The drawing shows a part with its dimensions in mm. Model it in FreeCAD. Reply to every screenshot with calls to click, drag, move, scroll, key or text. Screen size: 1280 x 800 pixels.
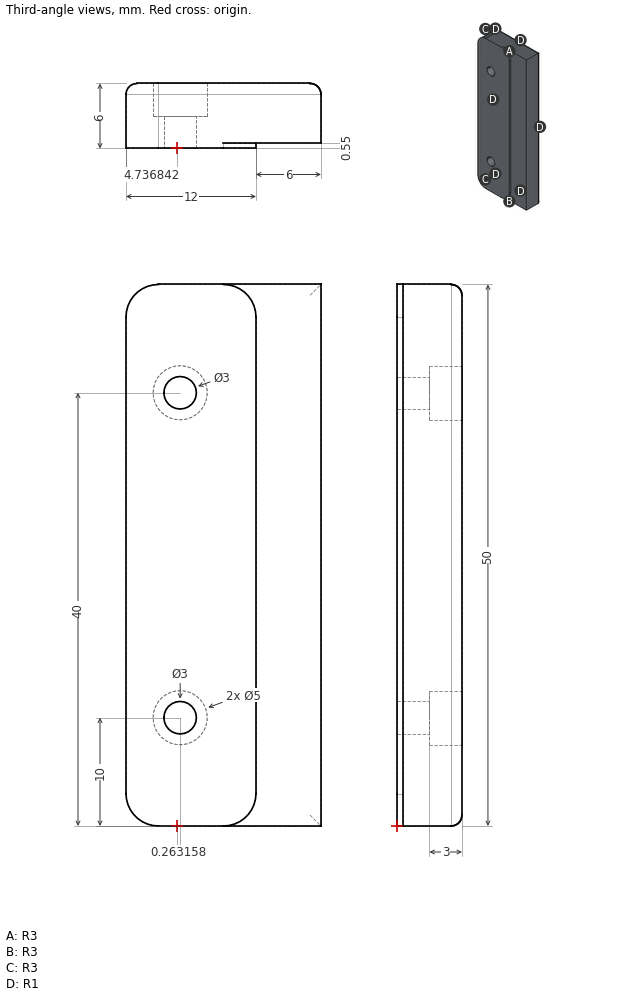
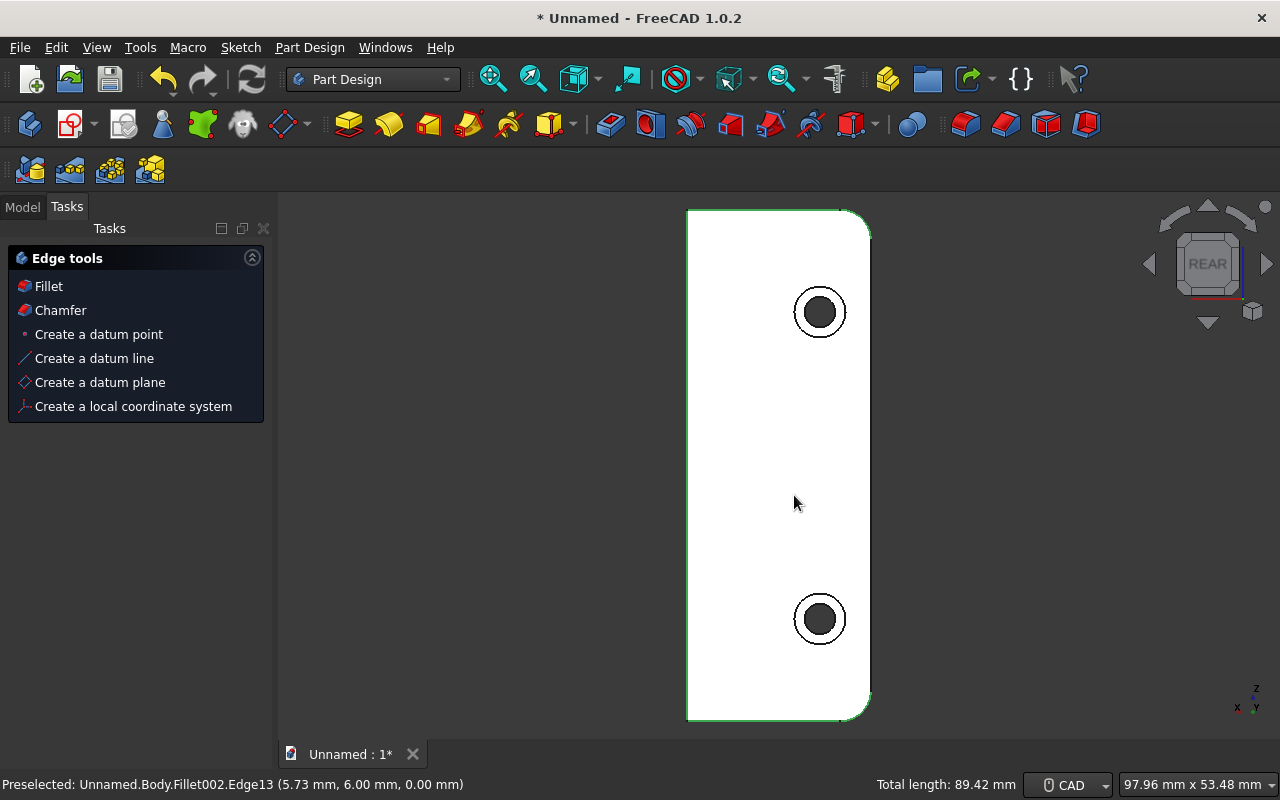
click(871, 464, ctrl)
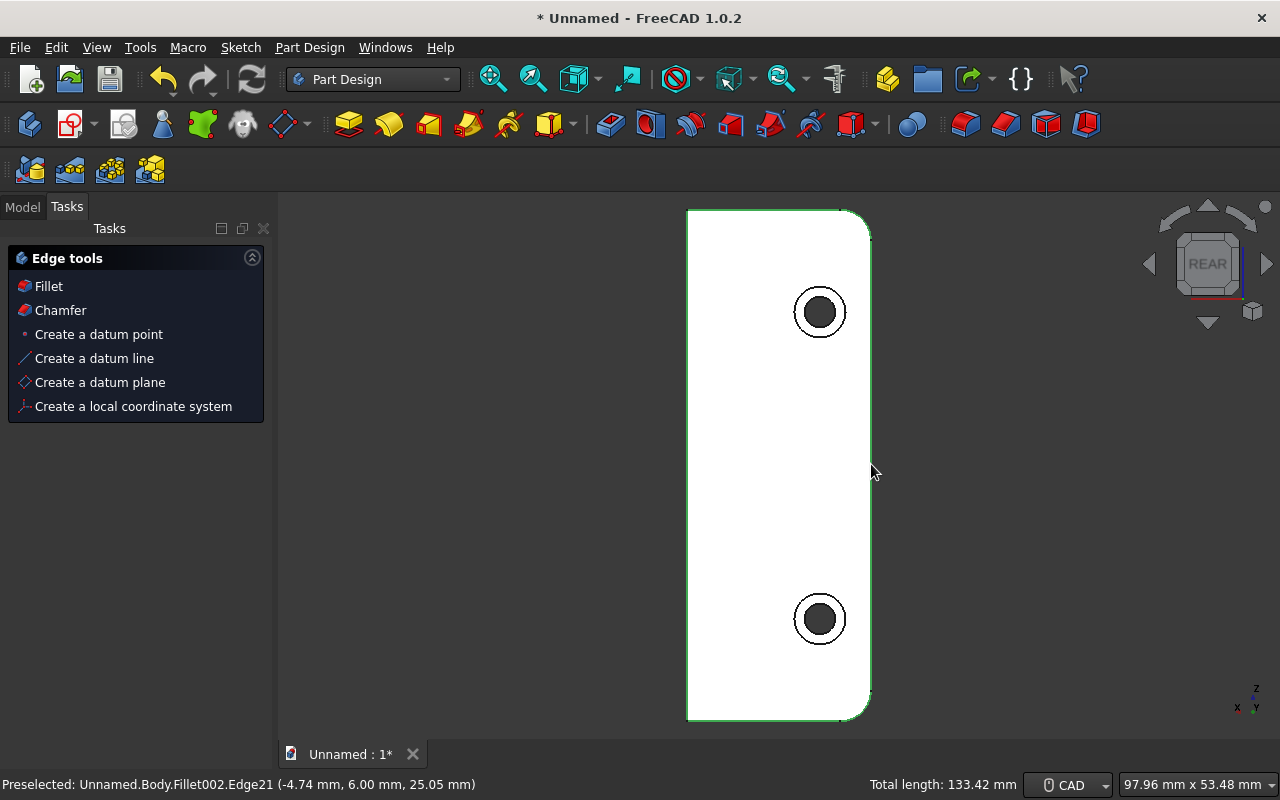
click(966, 124)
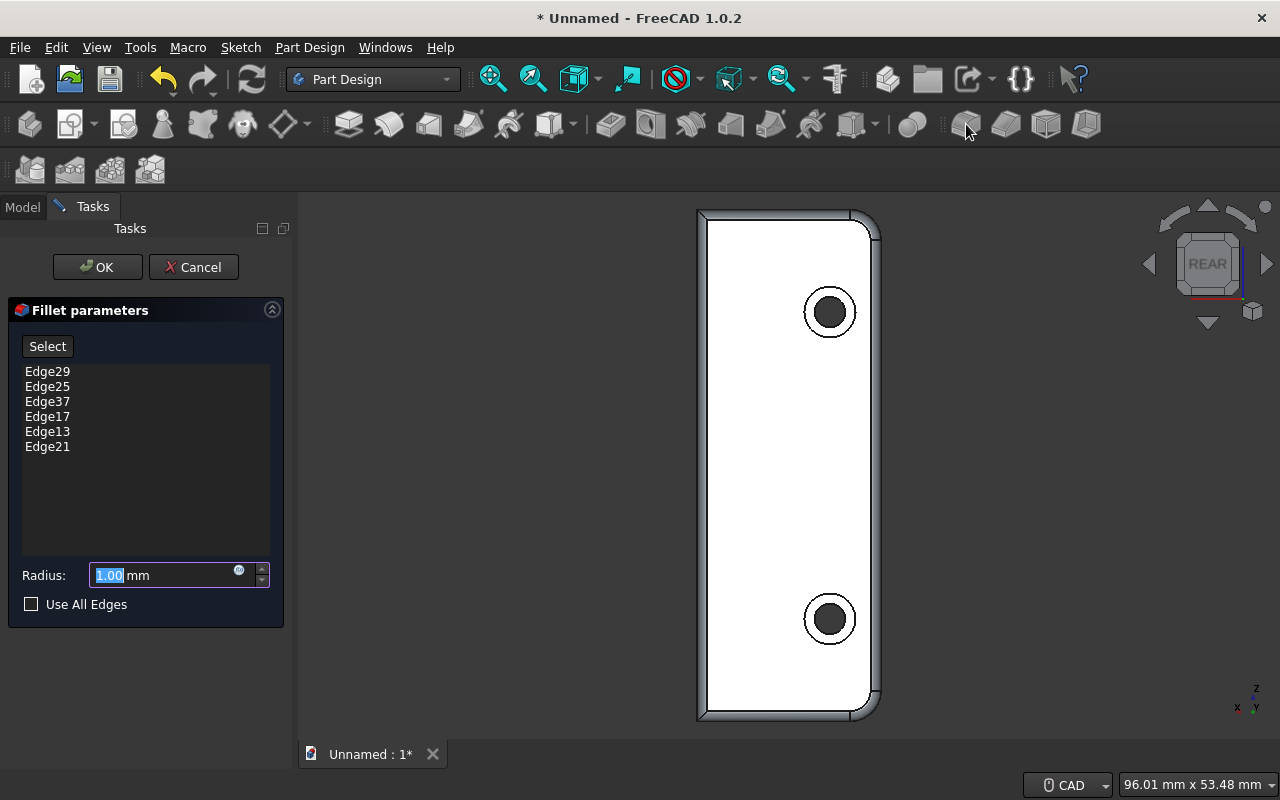
text(1)
key(Tab)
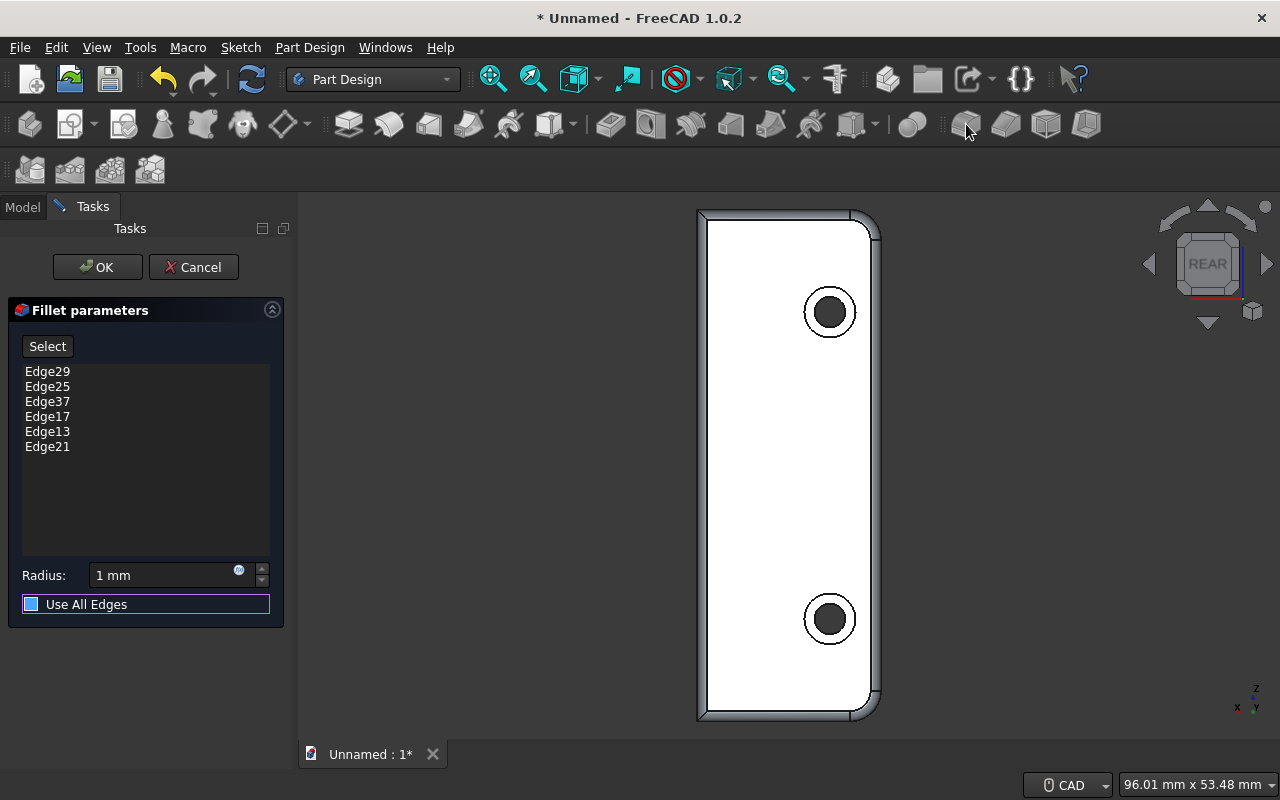
click(98, 267)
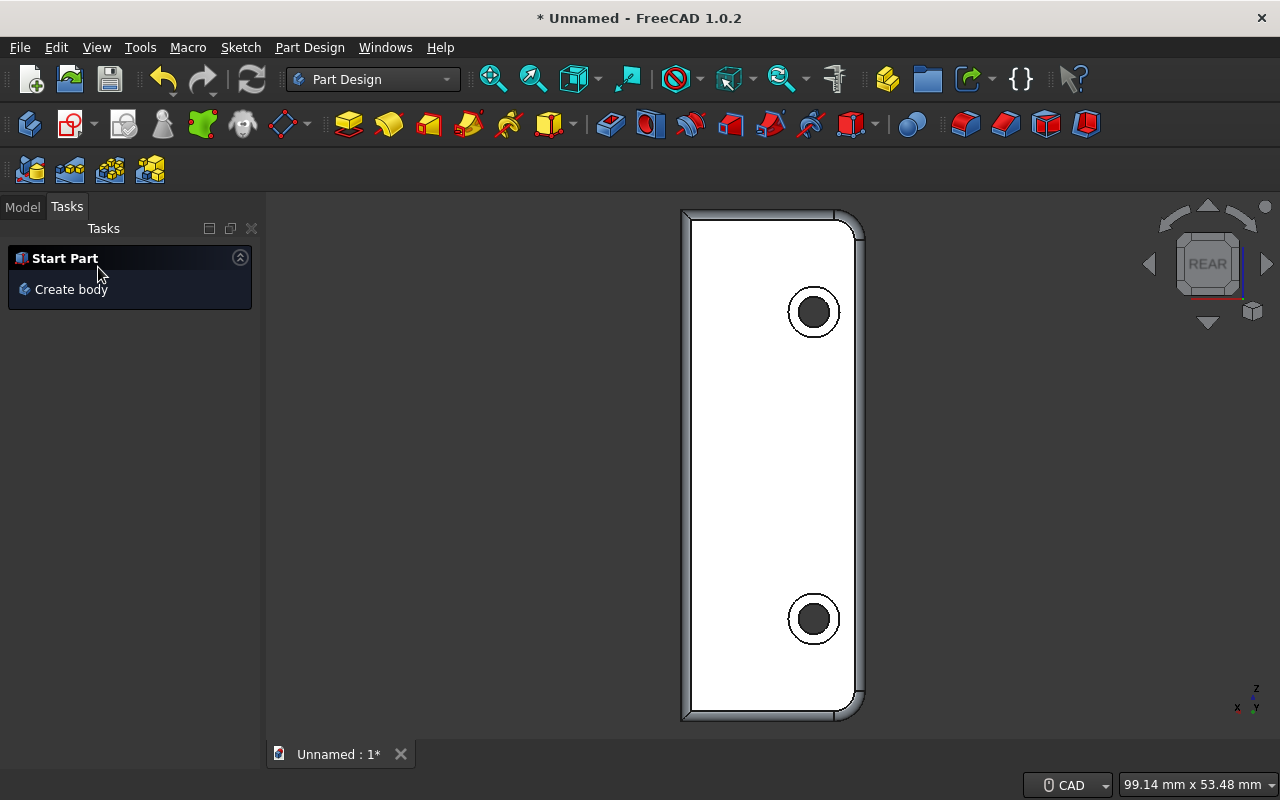
key(0)